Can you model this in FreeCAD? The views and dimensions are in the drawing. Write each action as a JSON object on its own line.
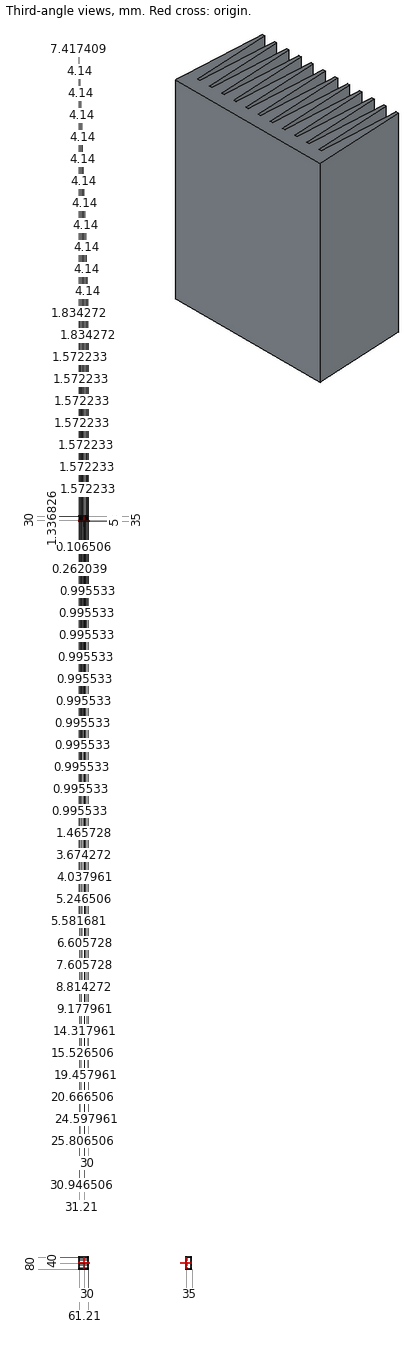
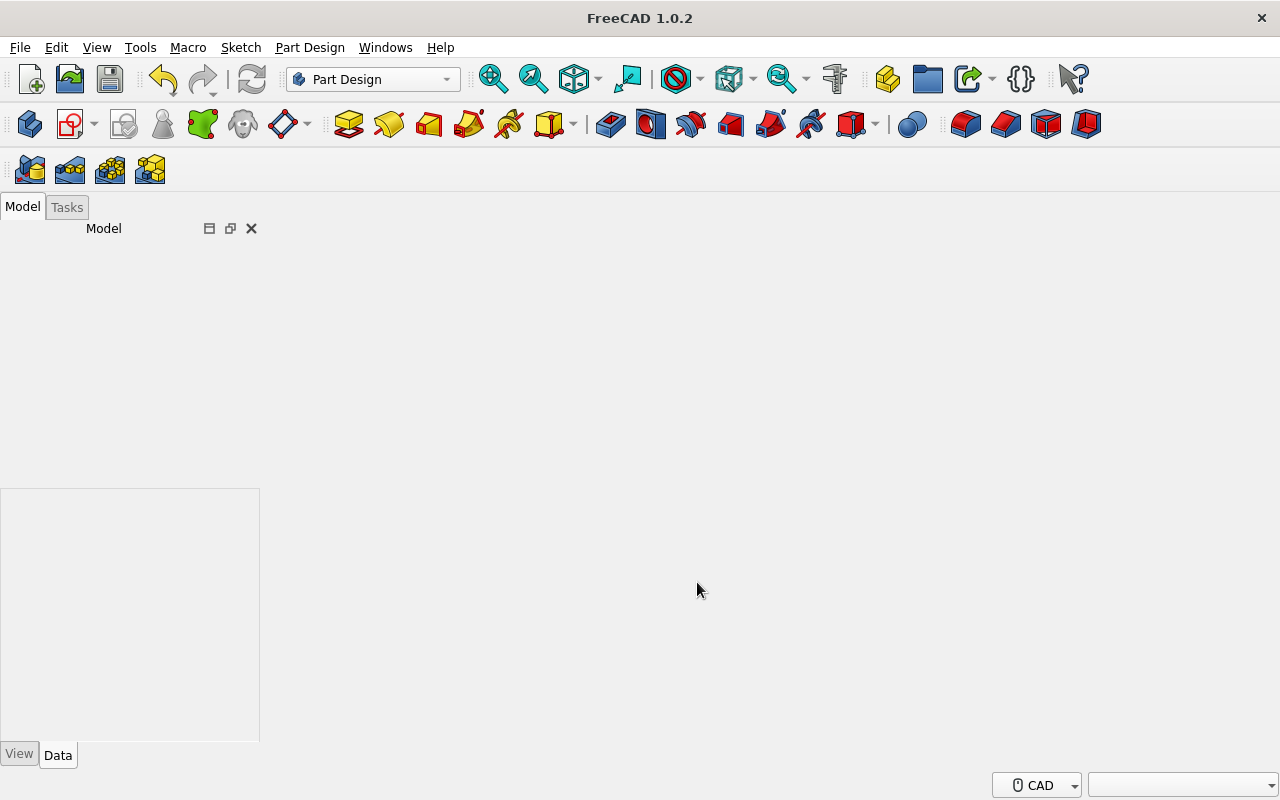
{"action": "left_click", "coordinate": [30, 80]}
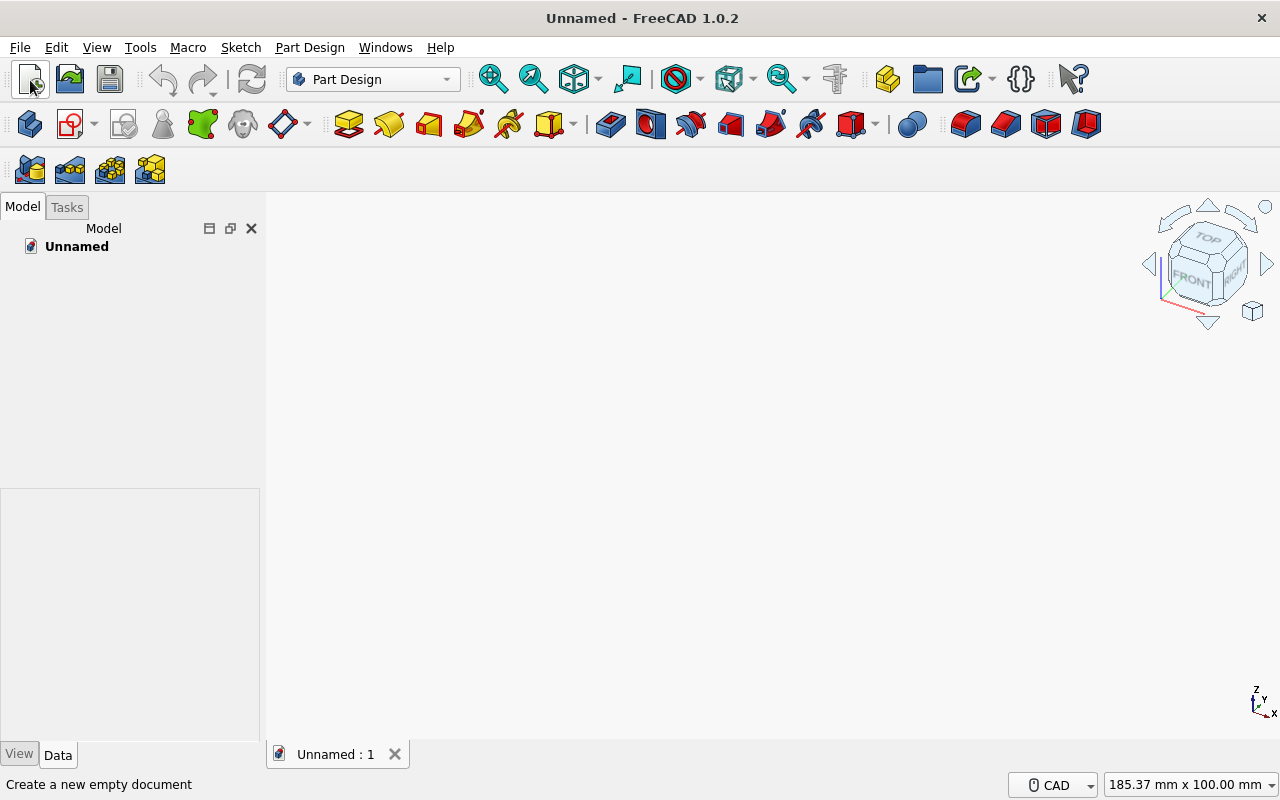
{"action": "left_click", "coordinate": [70, 124]}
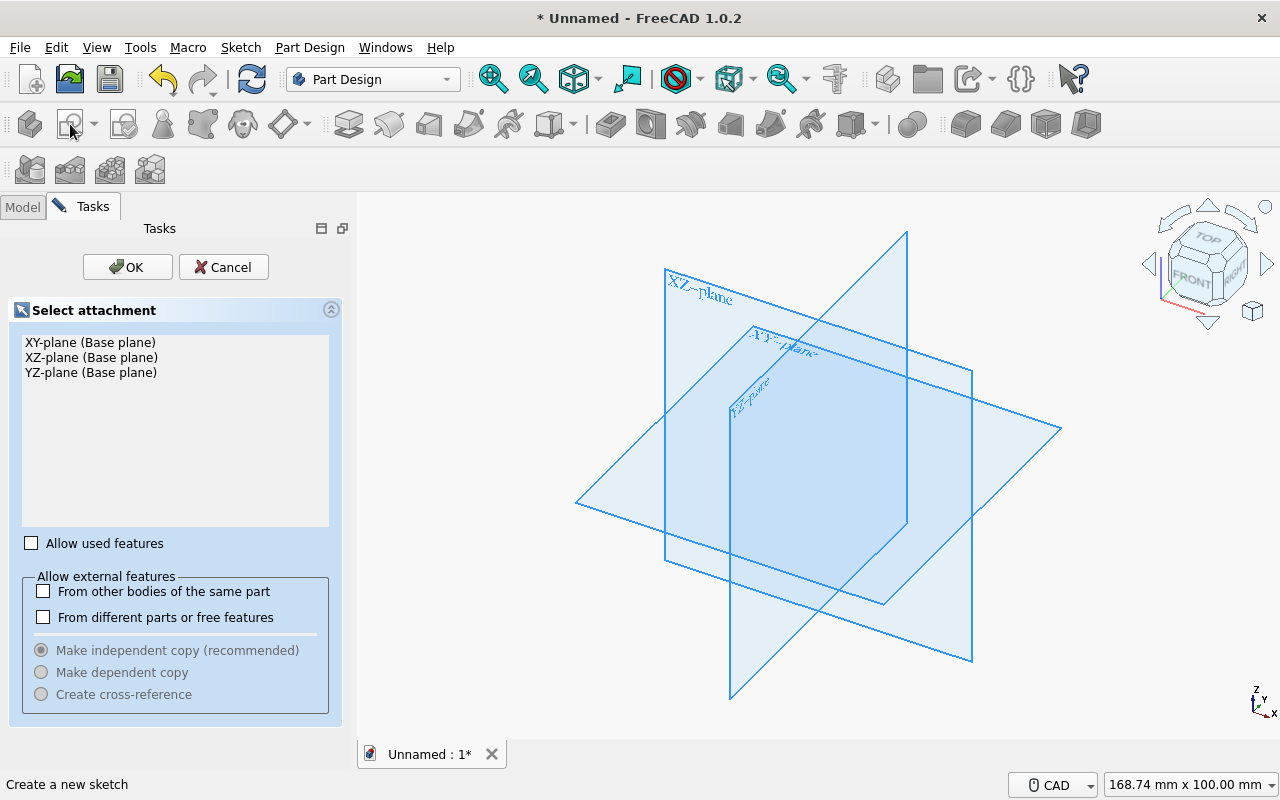
{"action": "left_click", "coordinate": [82, 358]}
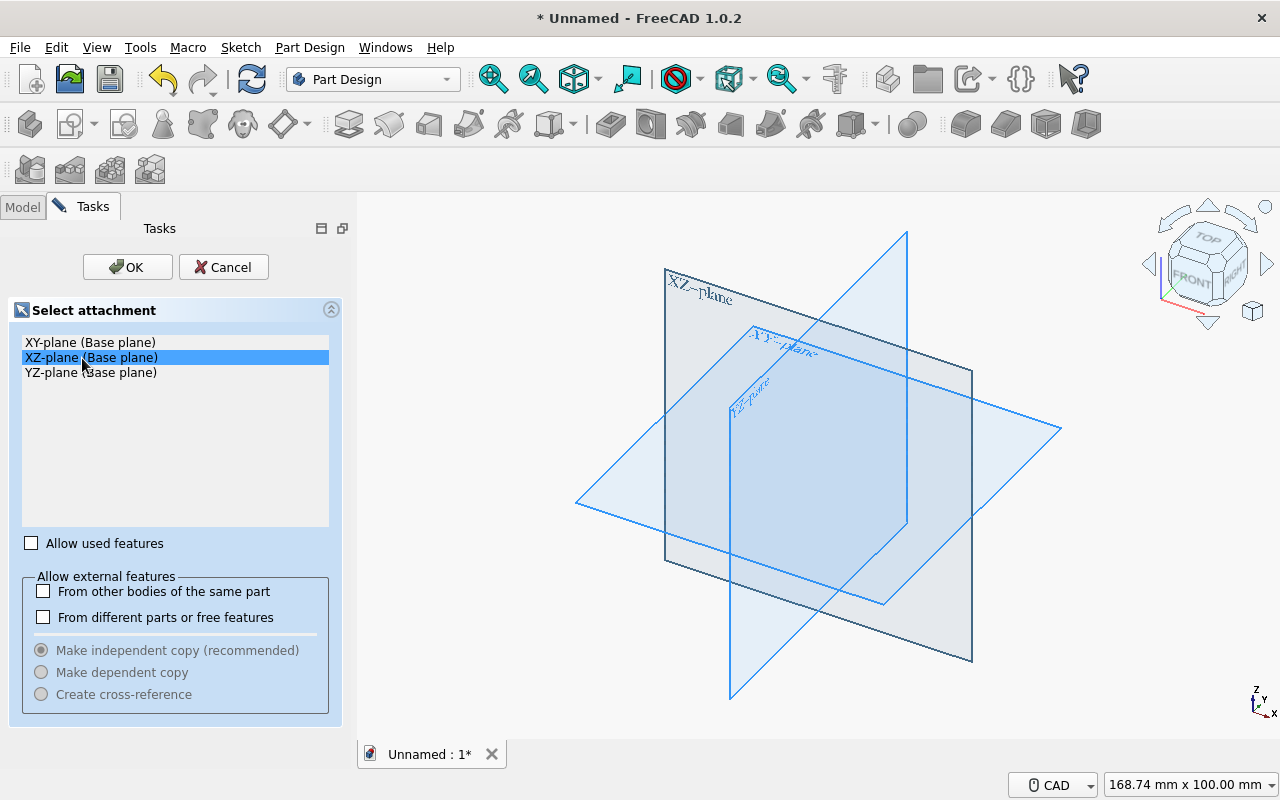
{"action": "left_click", "coordinate": [128, 267]}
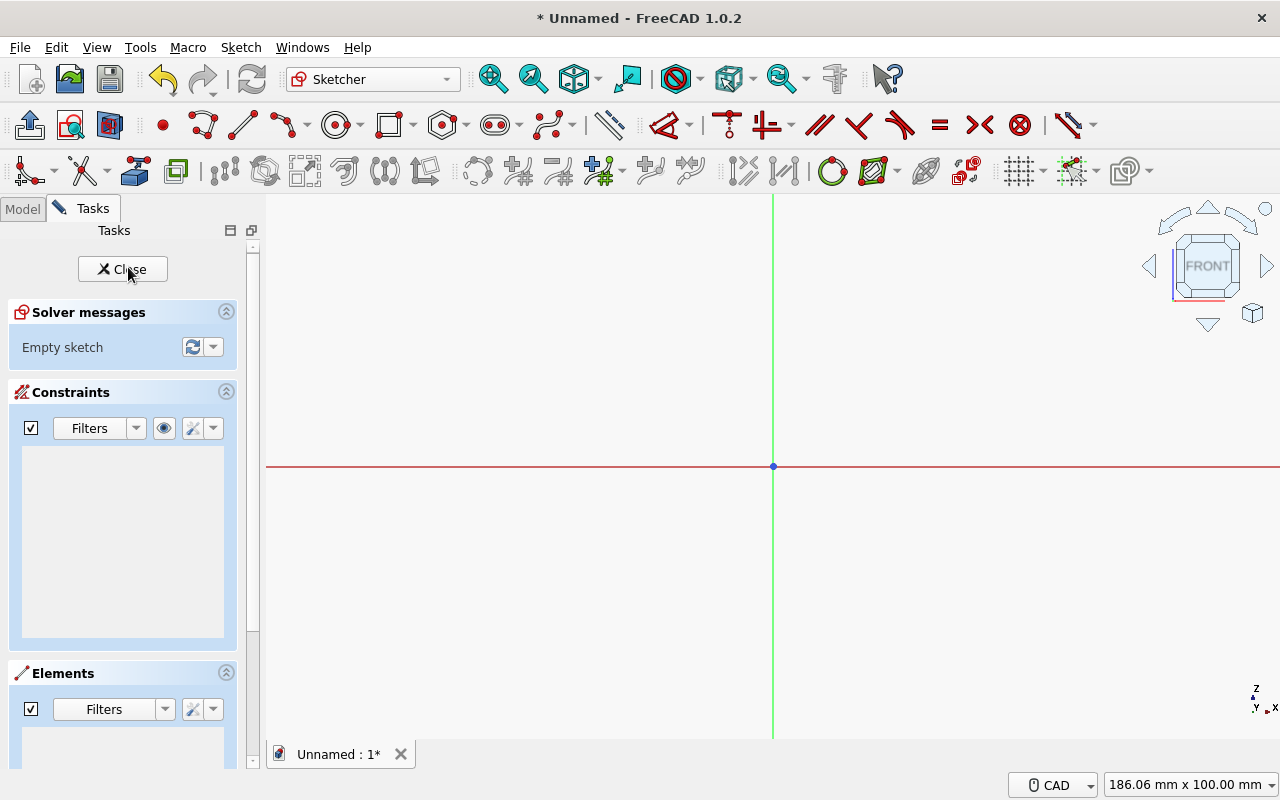
{"action": "left_click", "coordinate": [390, 126]}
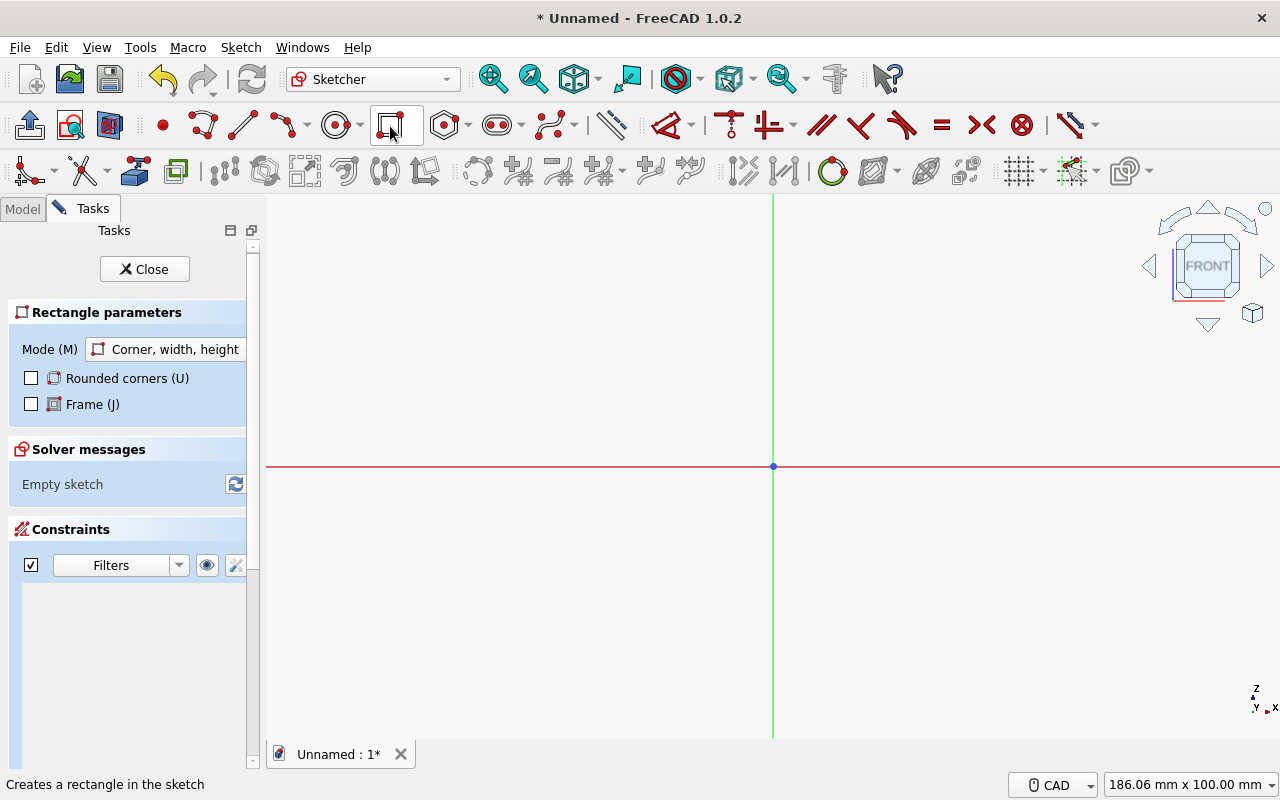
{"action": "left_click", "coordinate": [603, 249]}
{"action": "left_click", "coordinate": [936, 684]}
{"action": "key", "text": "Escape"}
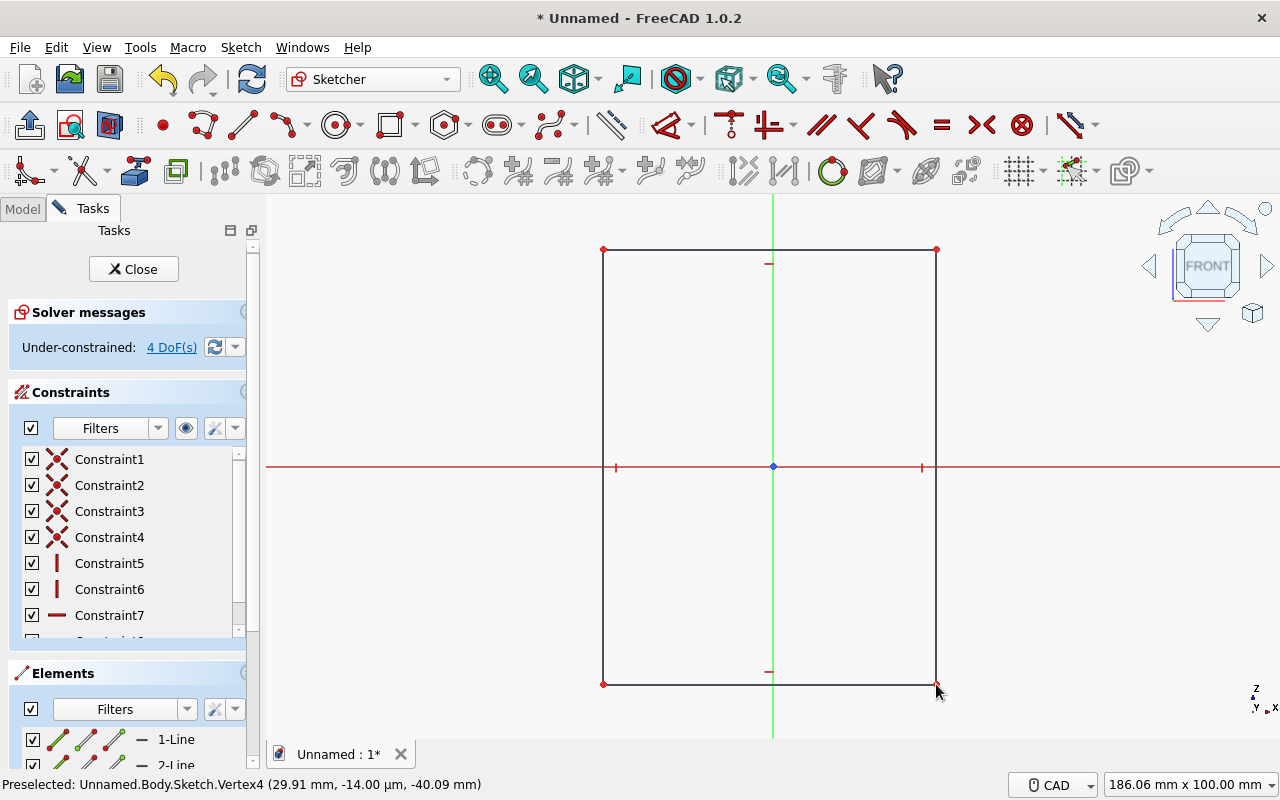
{"action": "left_click", "coordinate": [603, 380]}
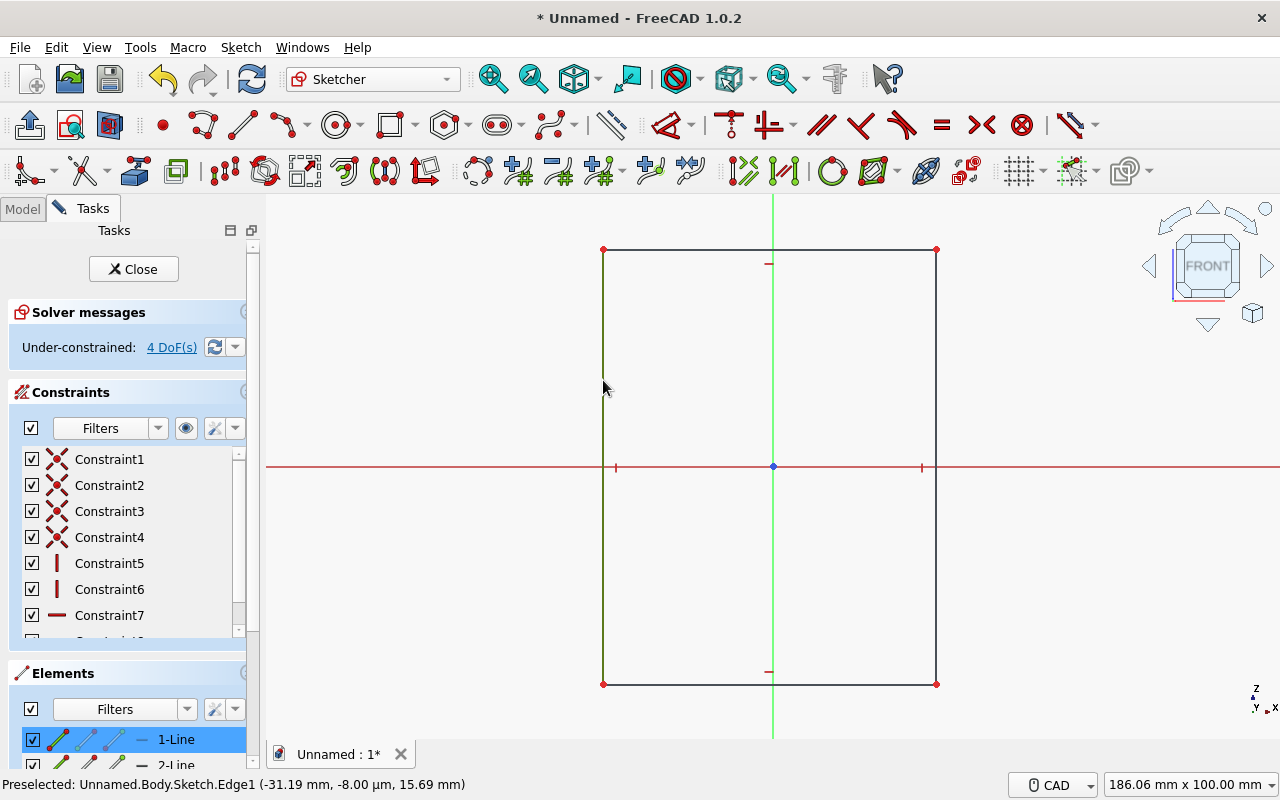
{"action": "left_click", "coordinate": [694, 126]}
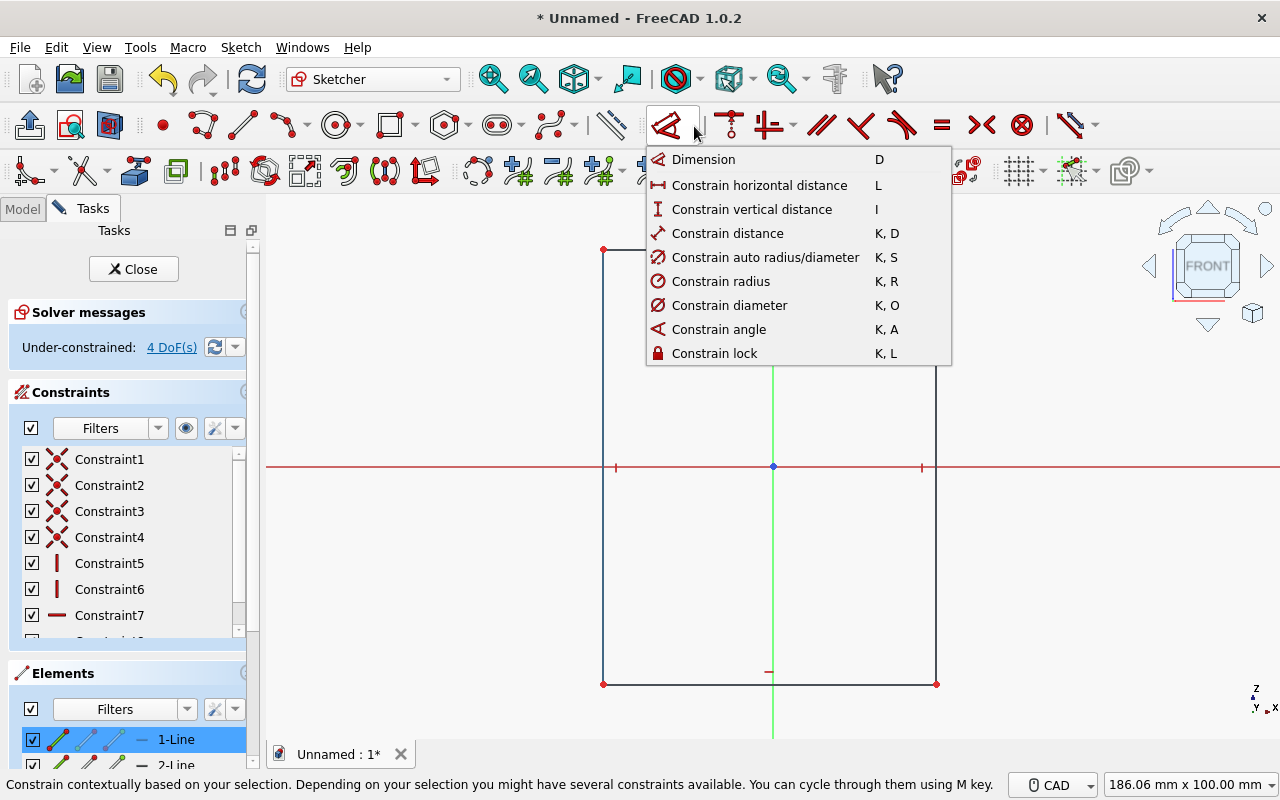
{"action": "left_click", "coordinate": [799, 209]}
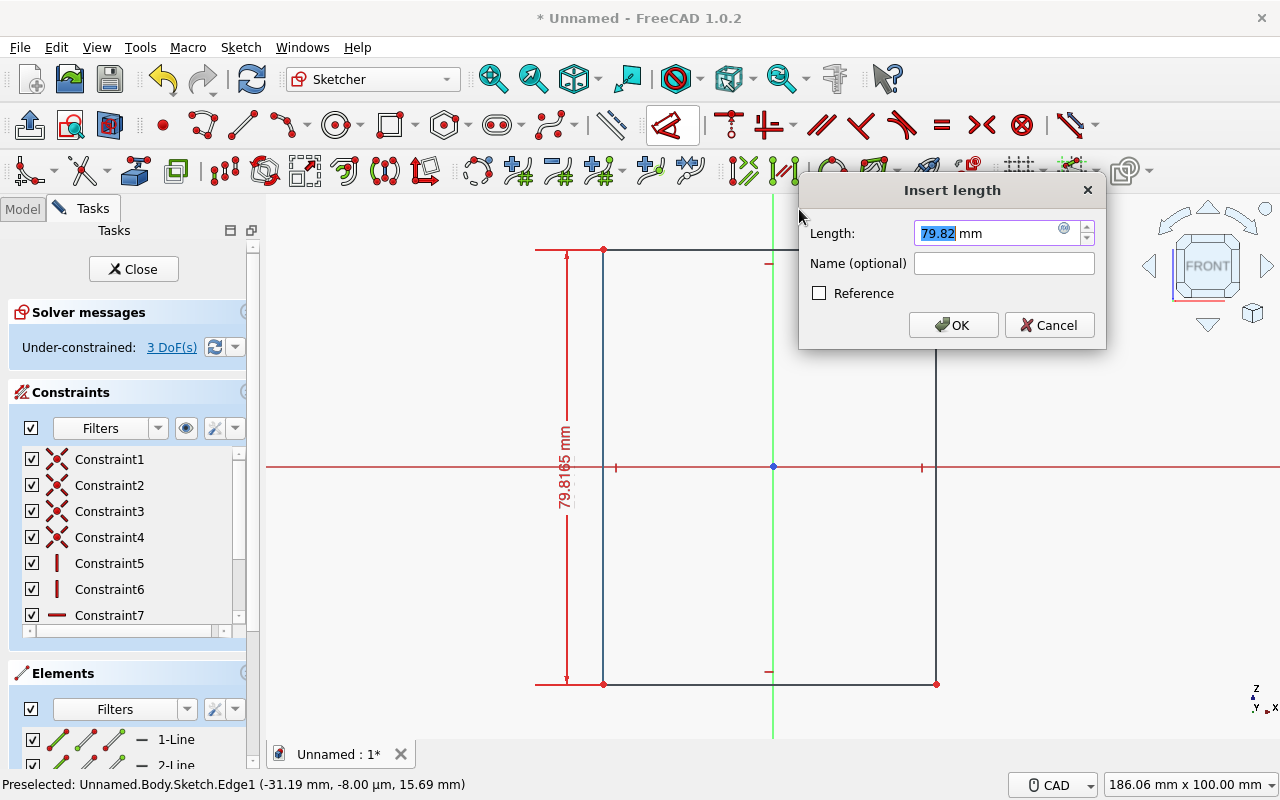
{"action": "type", "text": "80"}
{"action": "key", "text": "Return"}